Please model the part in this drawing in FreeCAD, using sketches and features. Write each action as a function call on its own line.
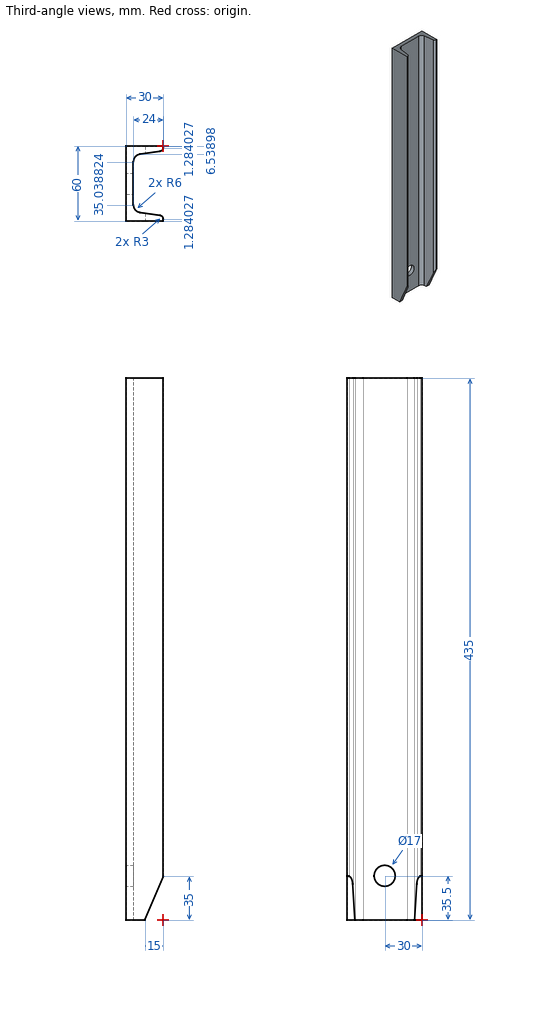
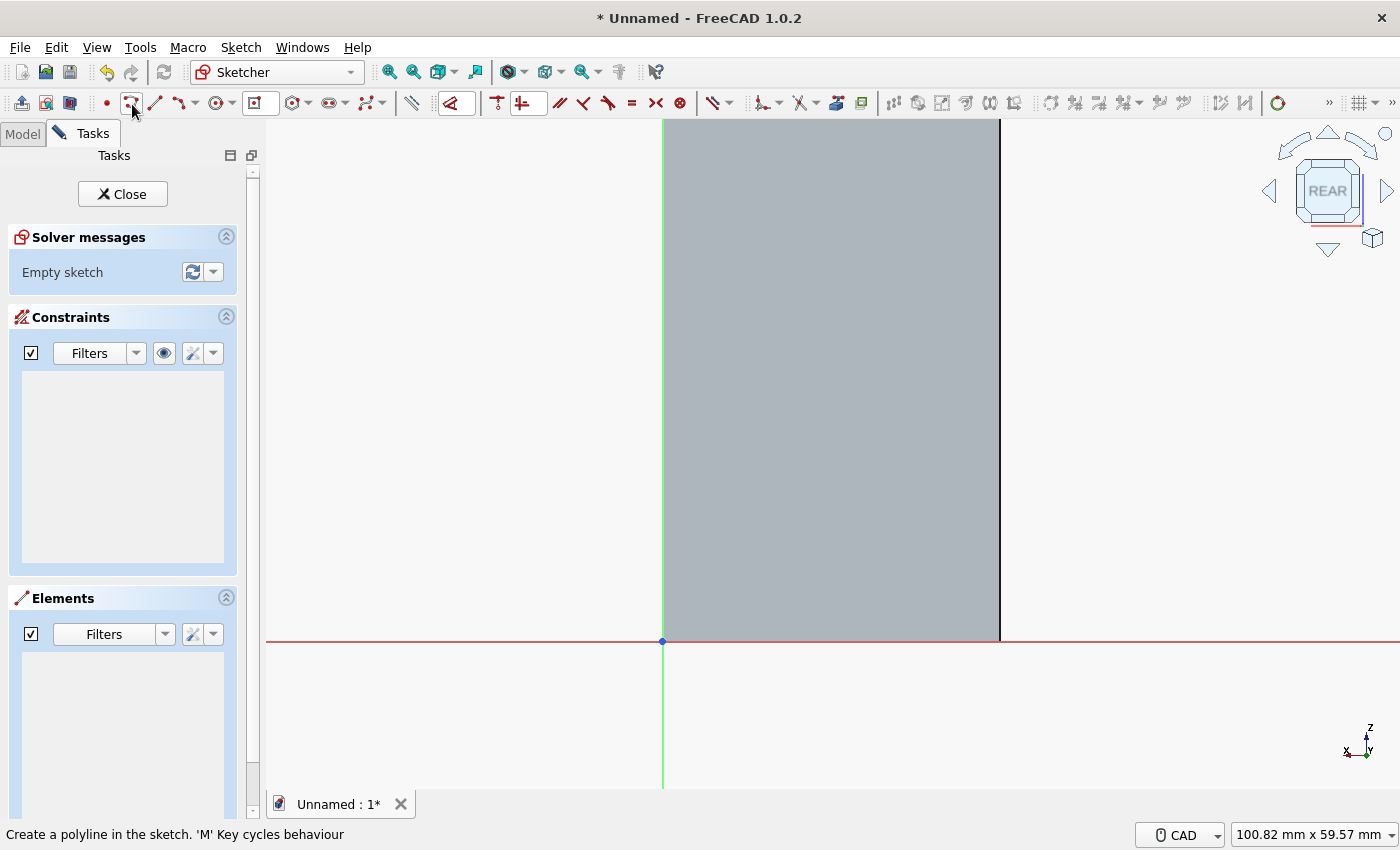
click(663, 642)
click(832, 633)
click(672, 248)
click(663, 642)
key(Escape)
key(Escape)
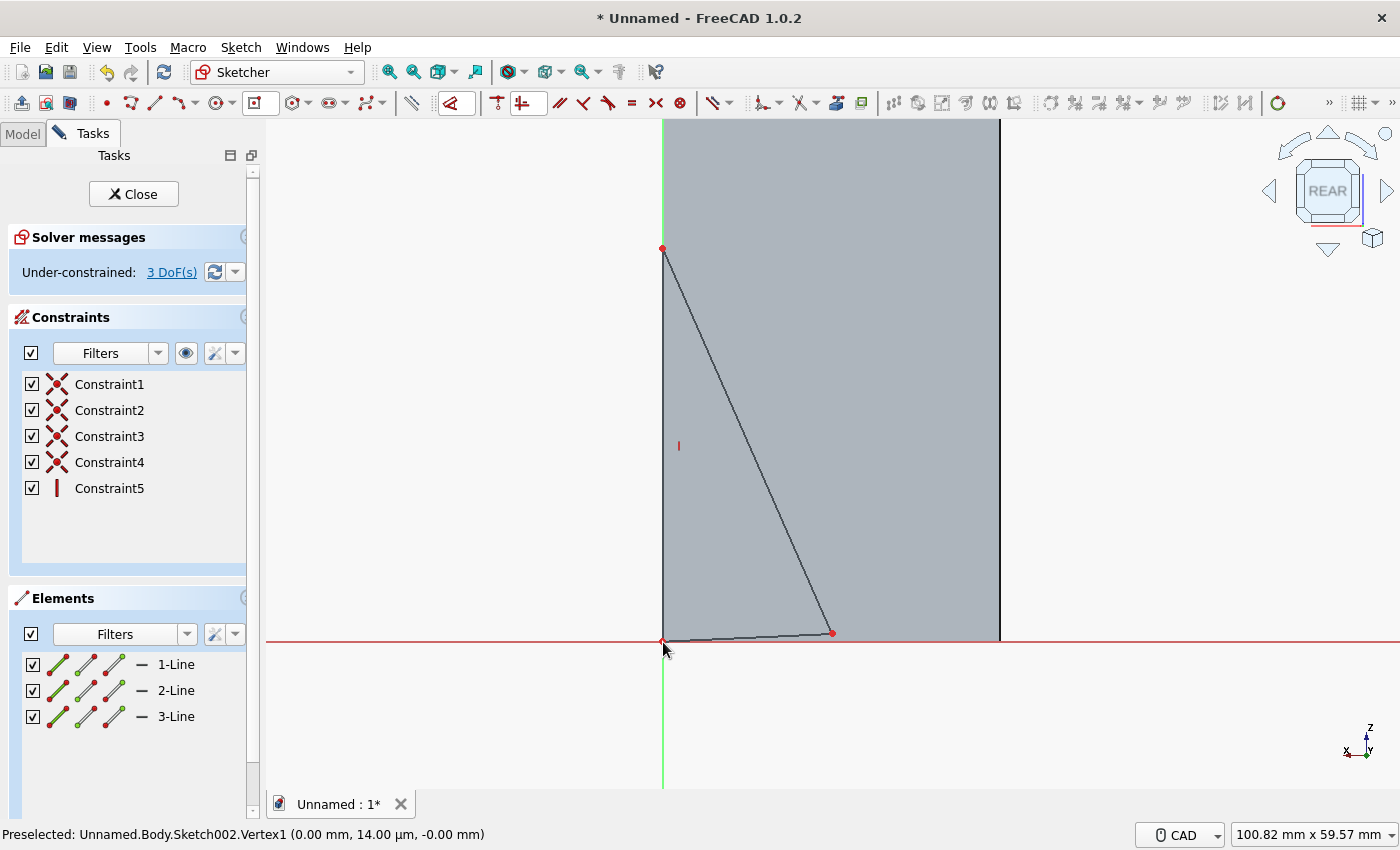
click(714, 639)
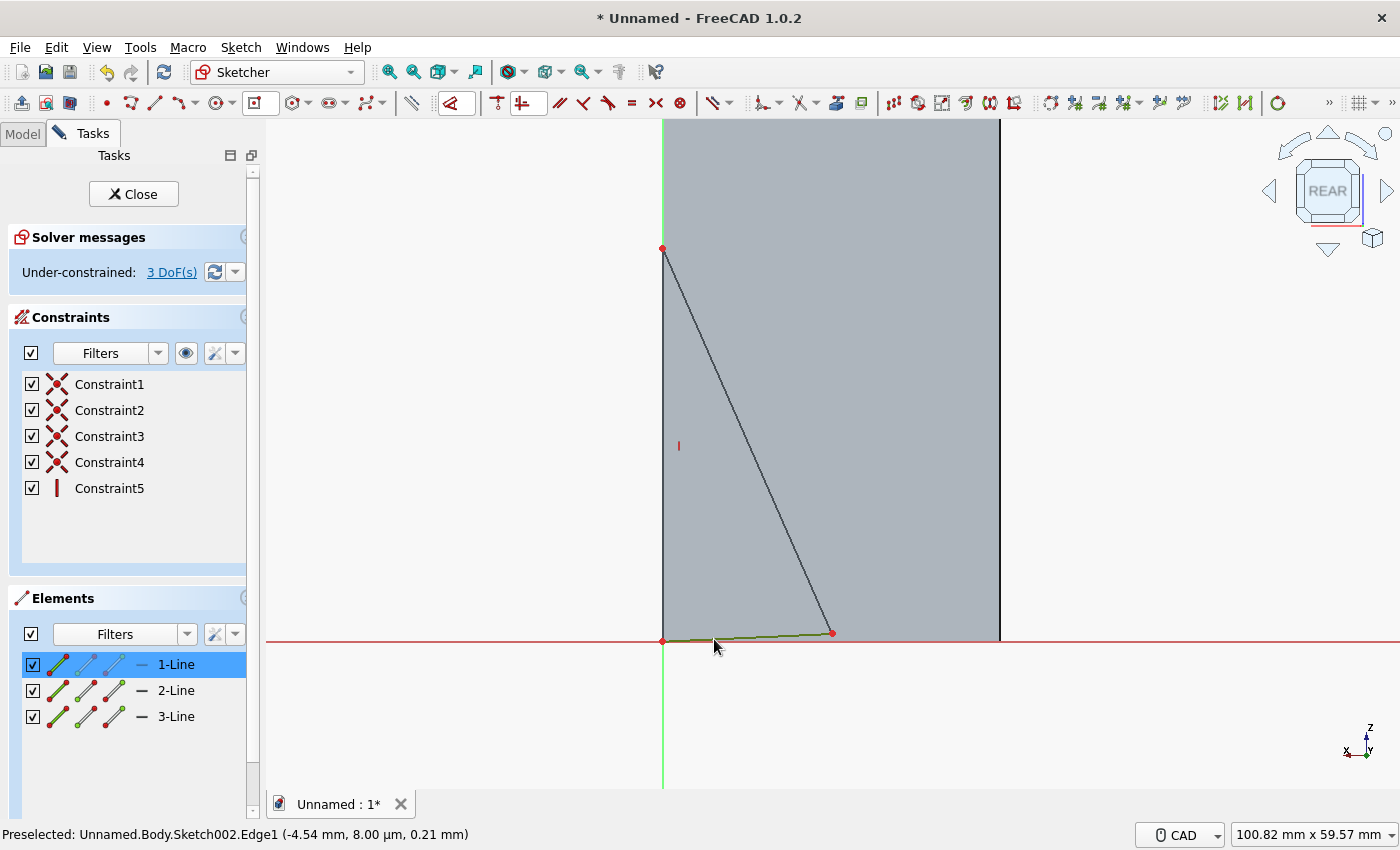
key(h)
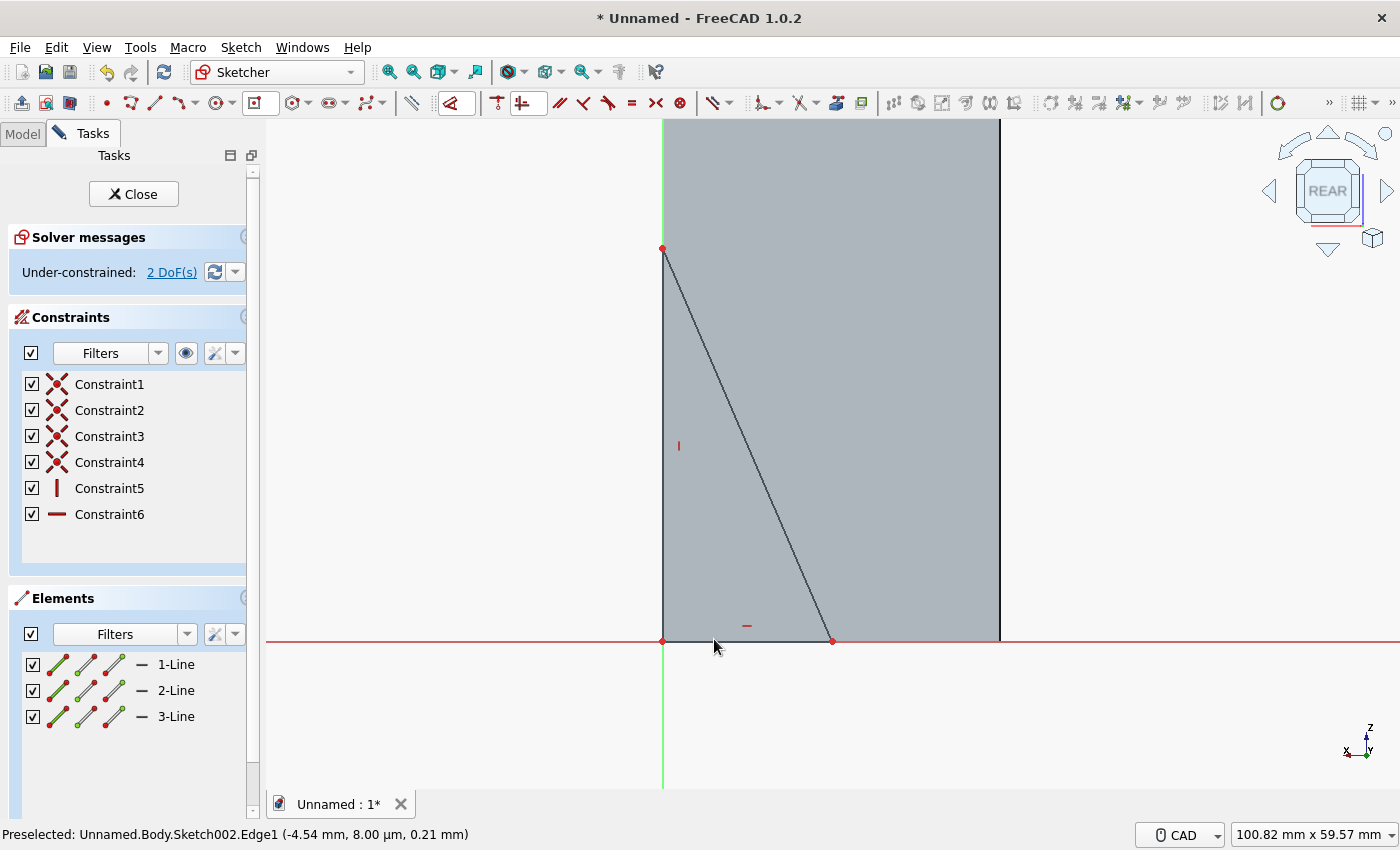
click(714, 642)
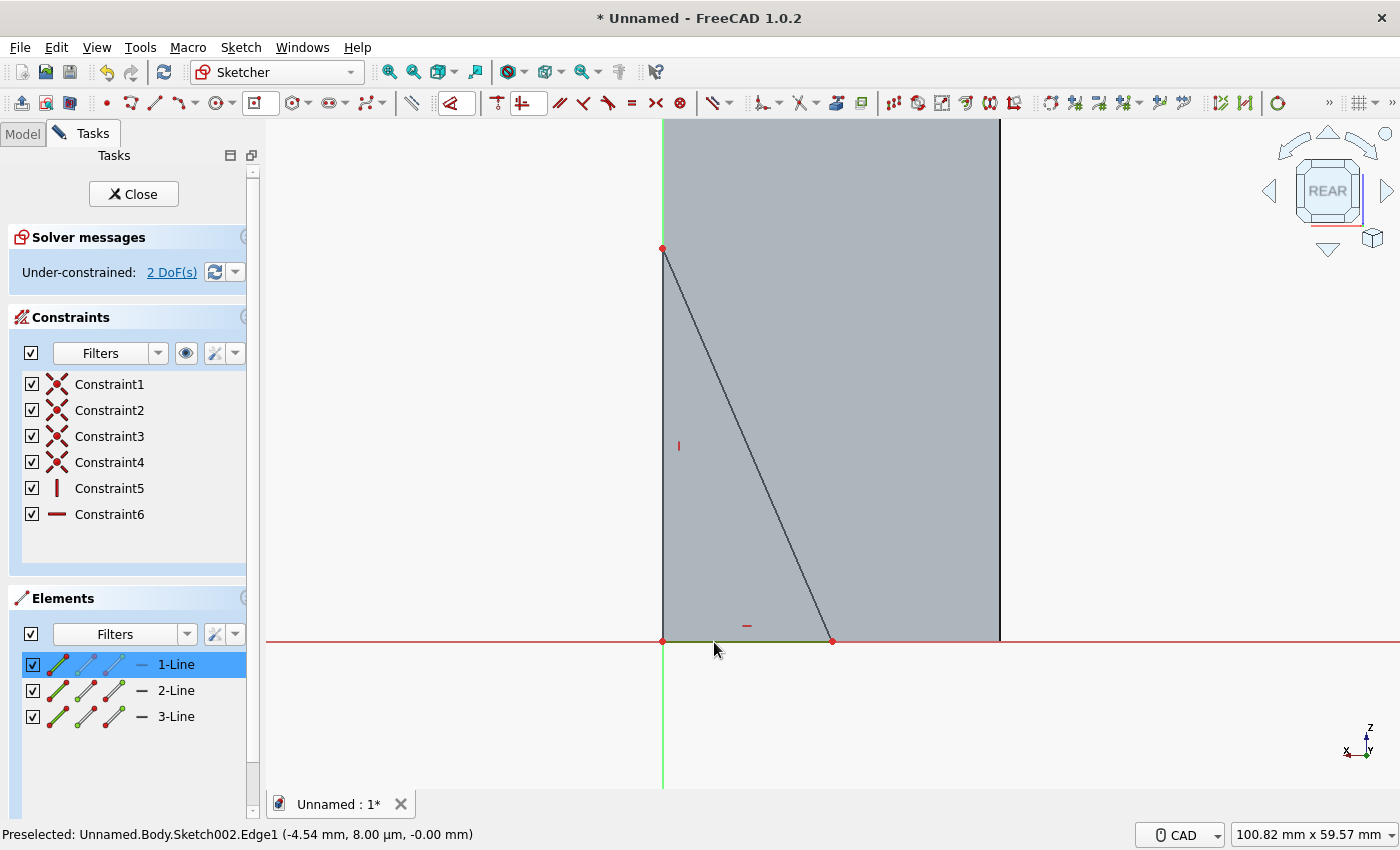
key(l)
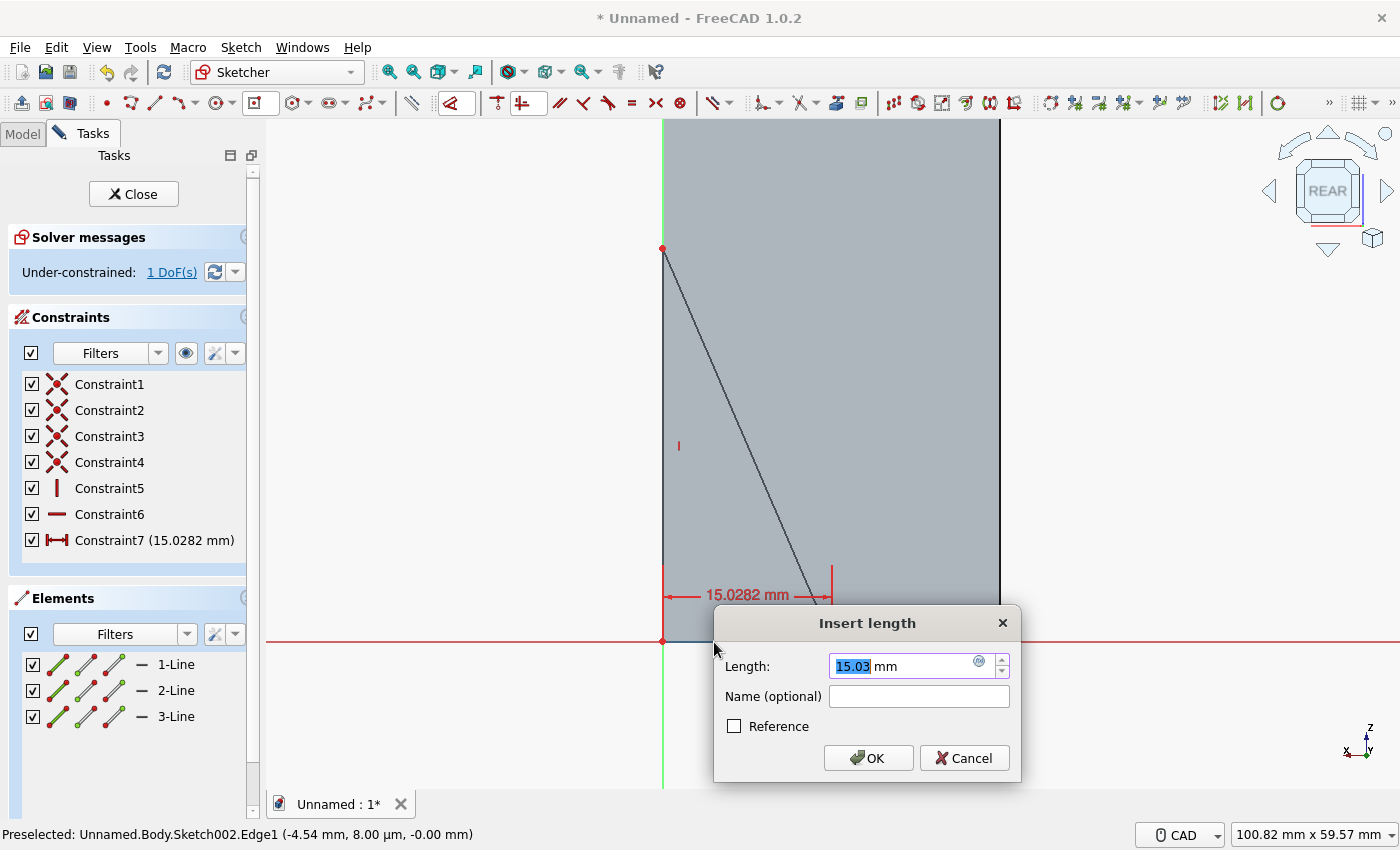
text(15)
key(Return)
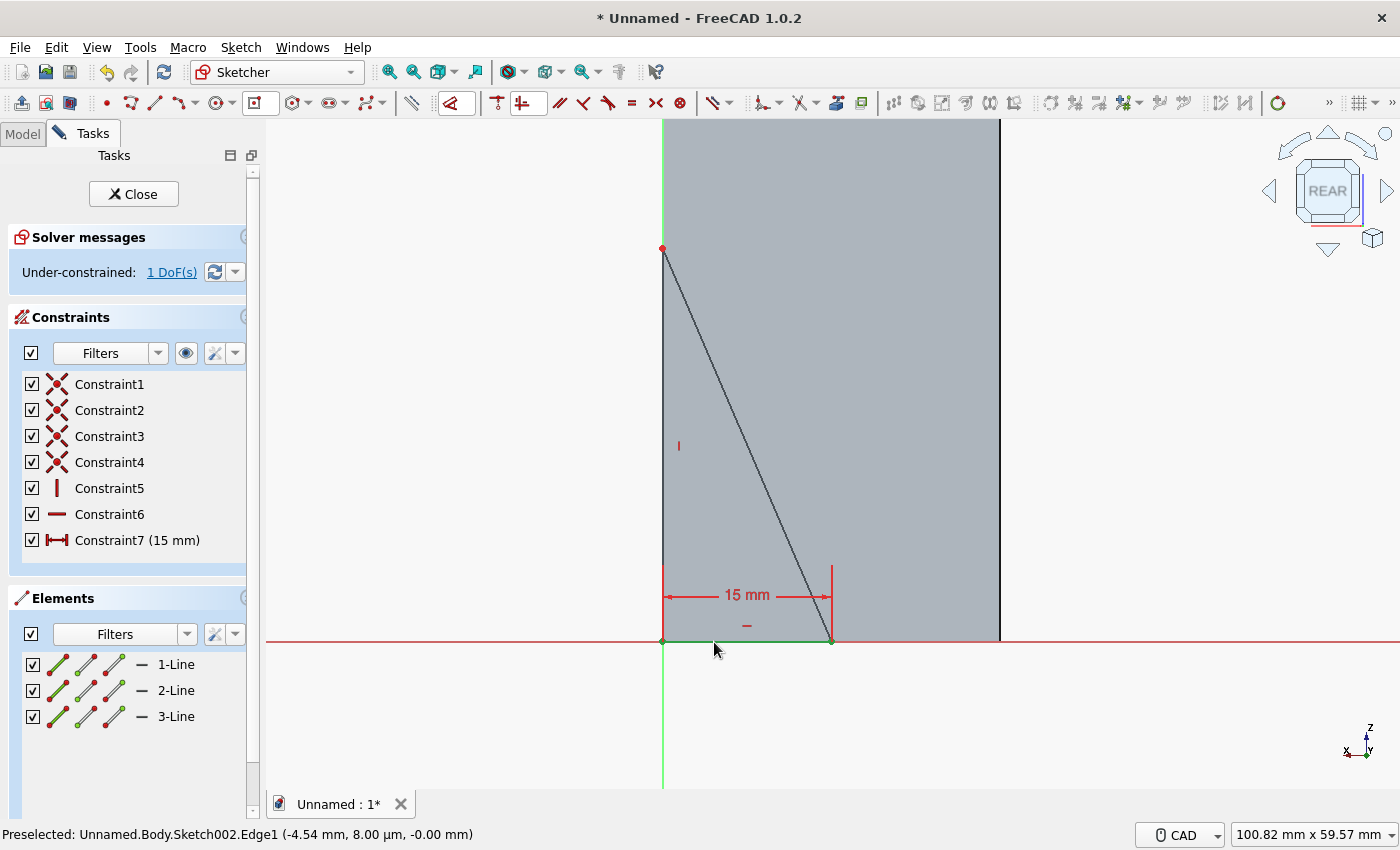
click(663, 367)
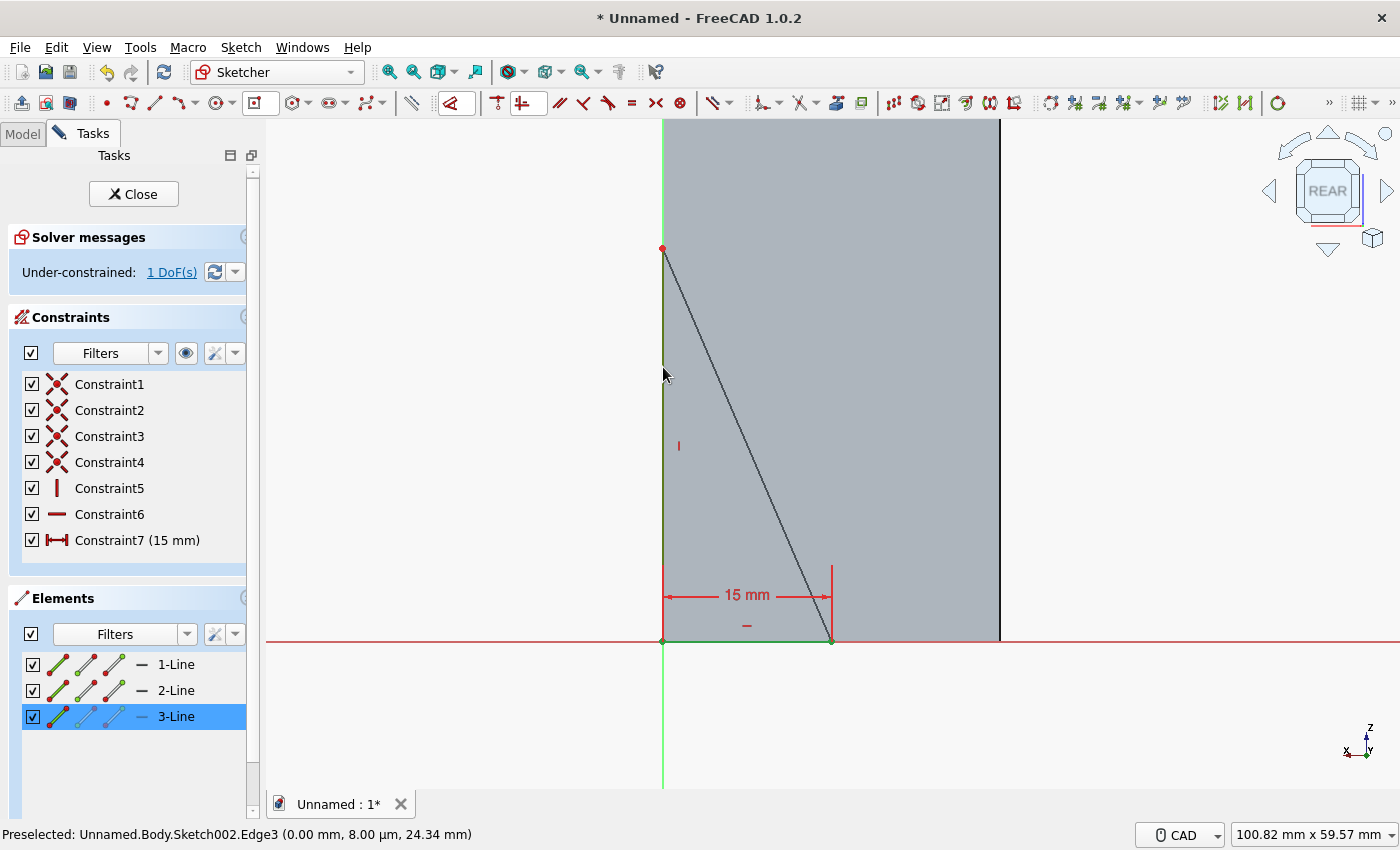
click(470, 104)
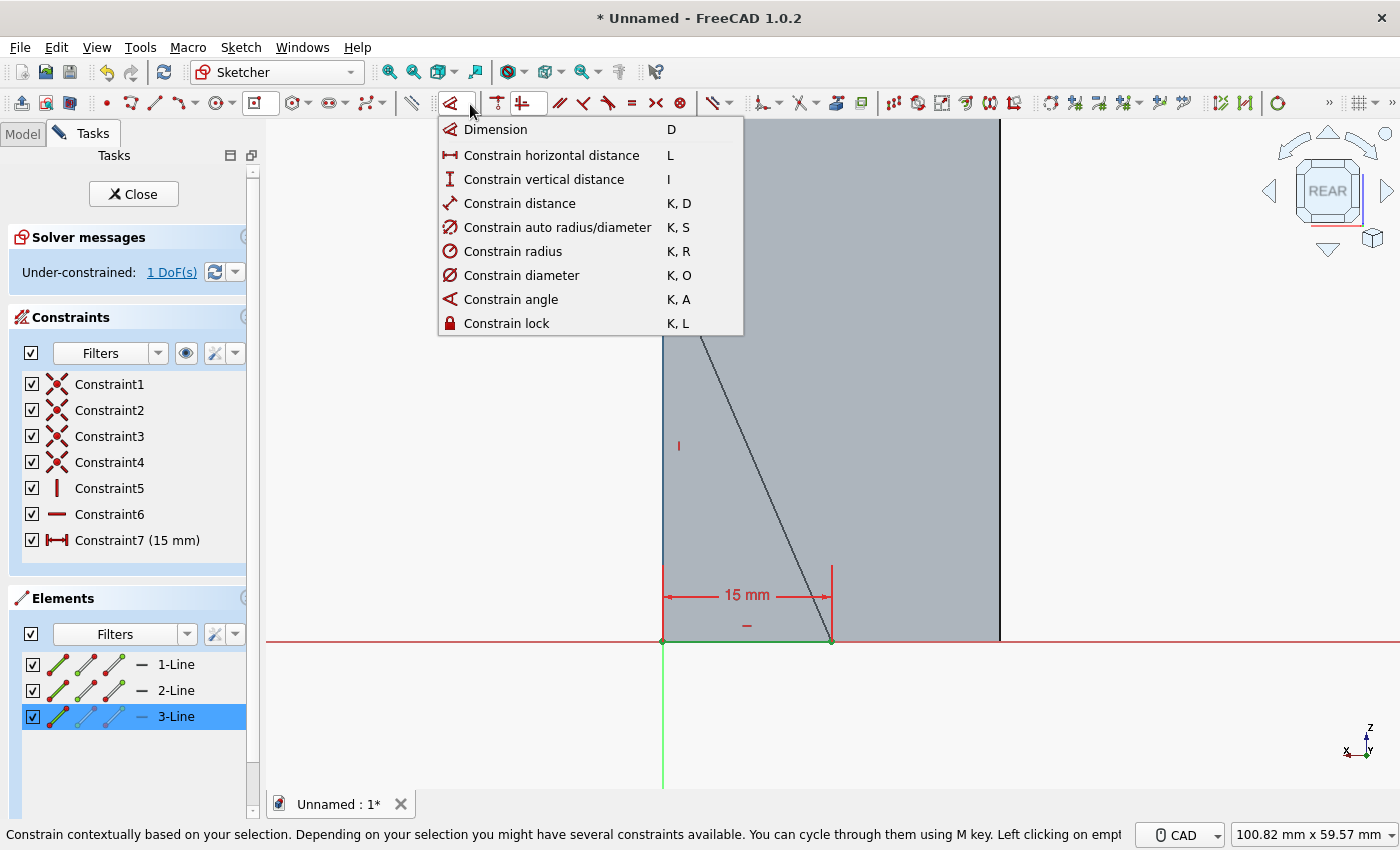
click(591, 179)